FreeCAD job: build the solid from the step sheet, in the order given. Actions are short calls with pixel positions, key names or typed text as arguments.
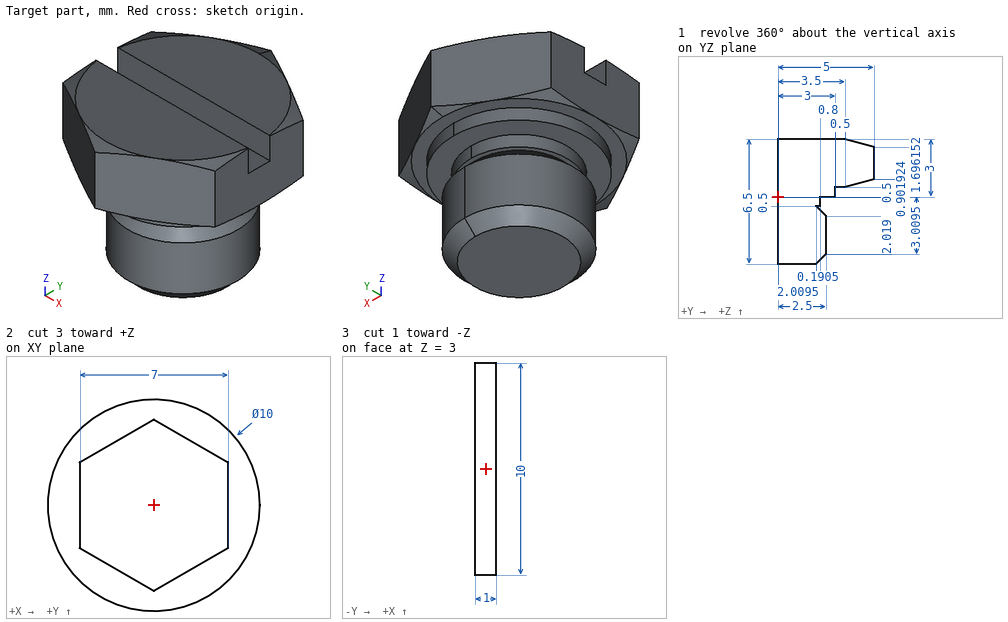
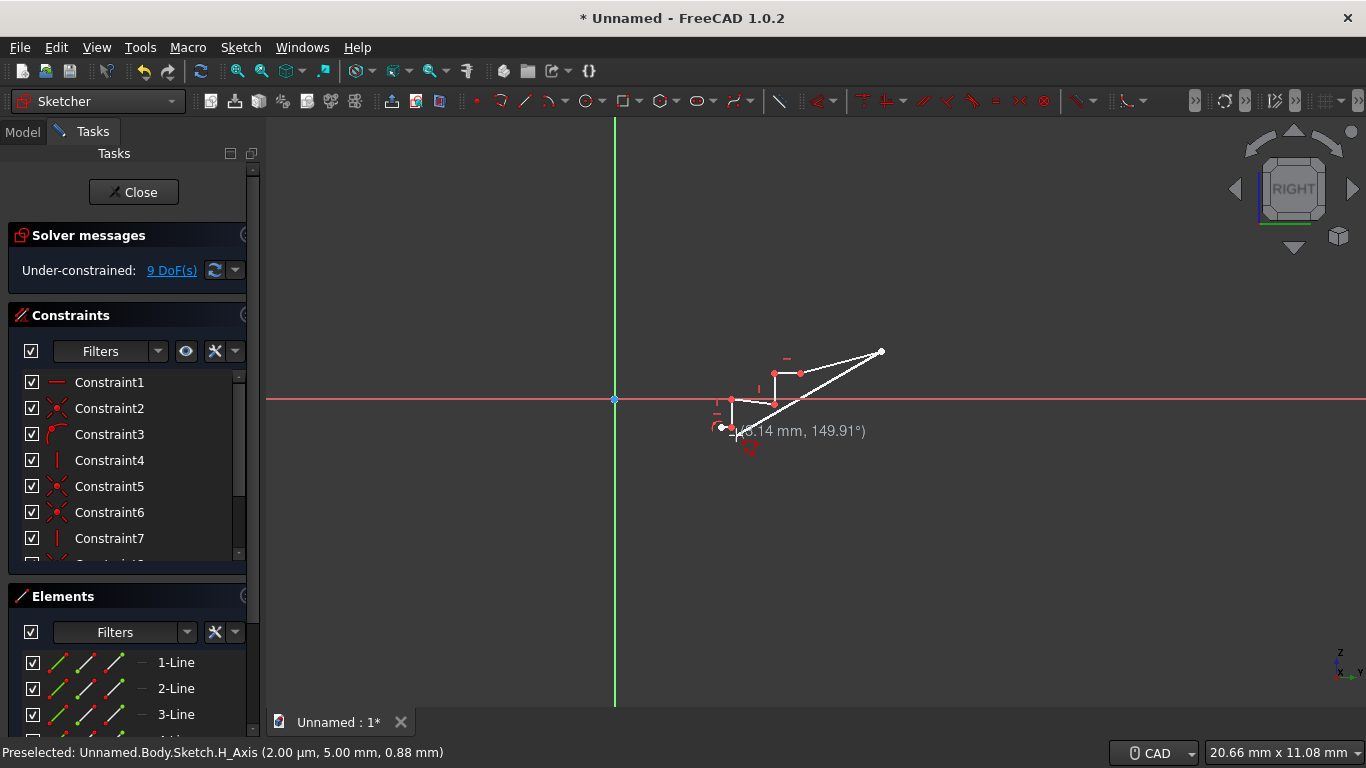
click(881, 261)
click(801, 239)
click(615, 239)
click(624, 586)
click(722, 586)
click(748, 559)
click(748, 452)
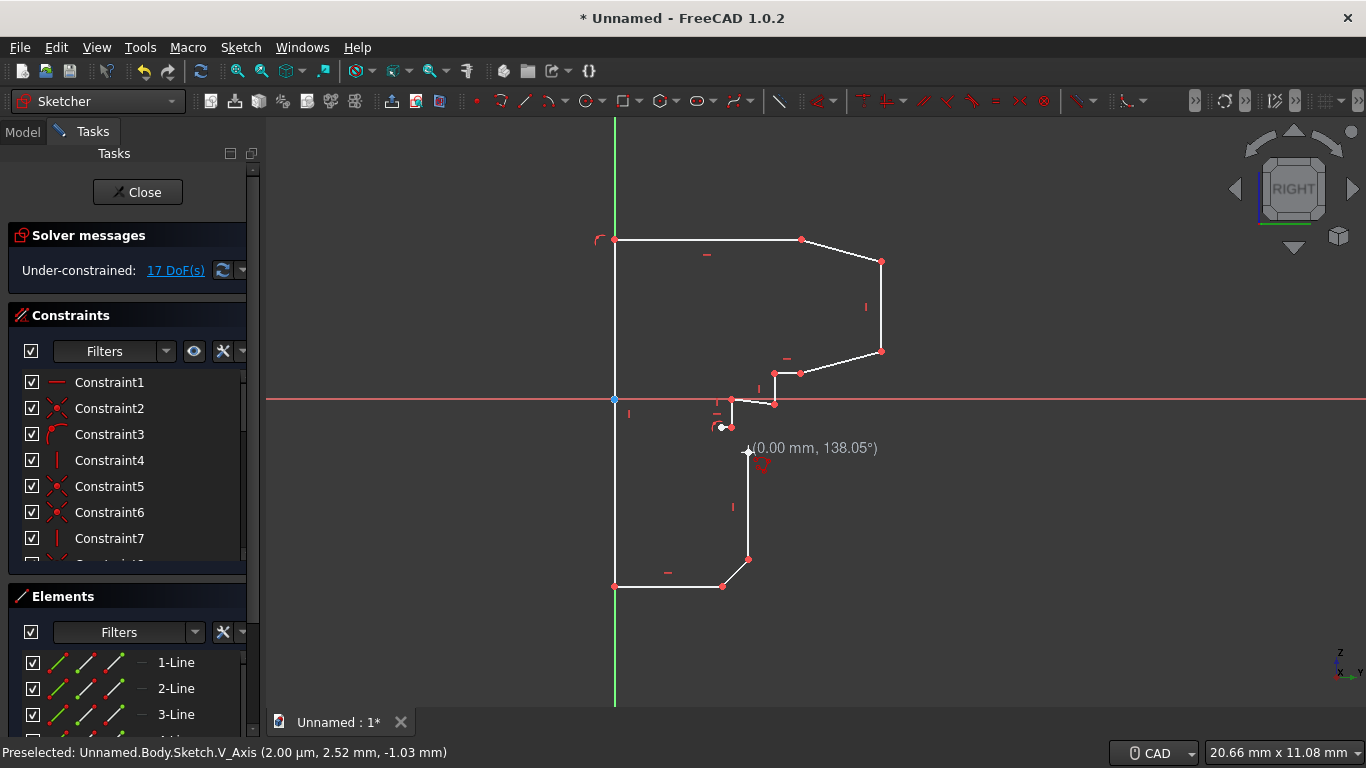
scroll(722, 426, up, 6)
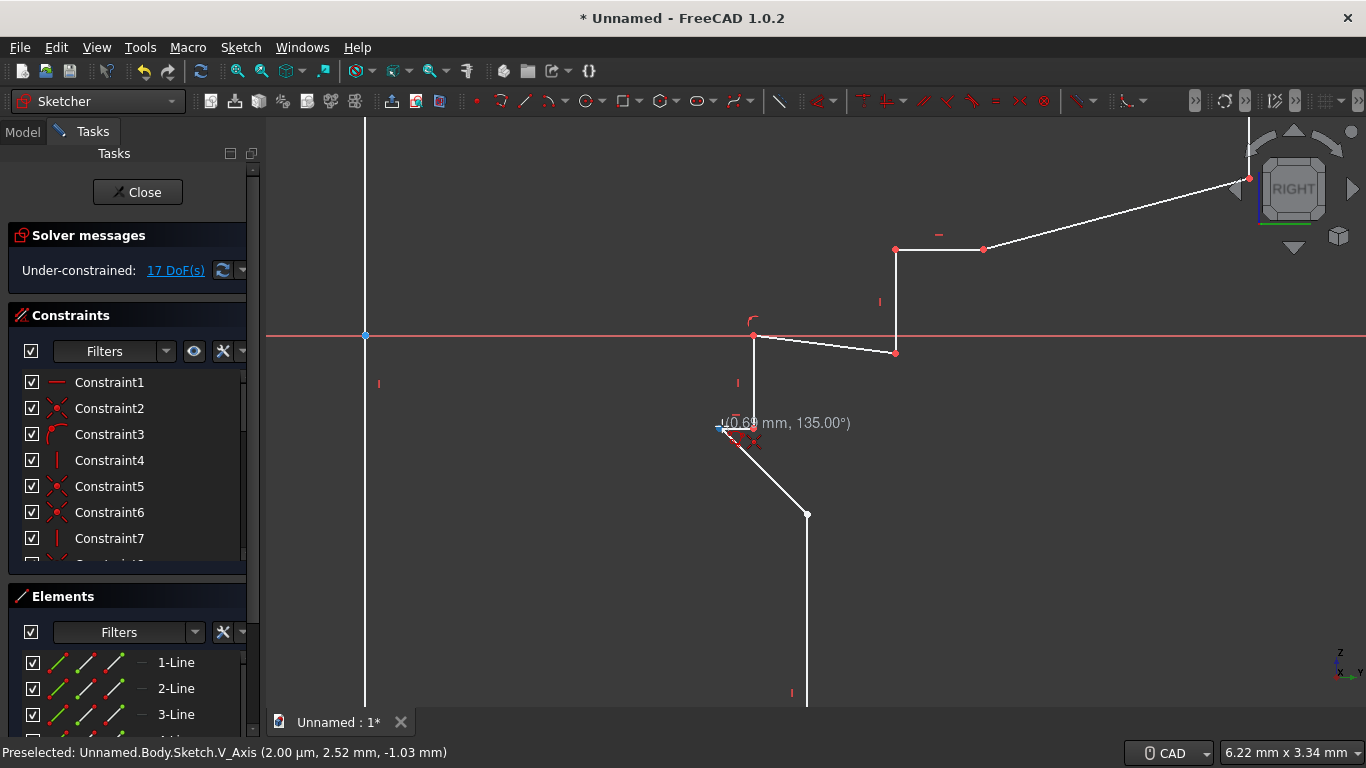
click(720, 429)
key(Escape)
key(Escape)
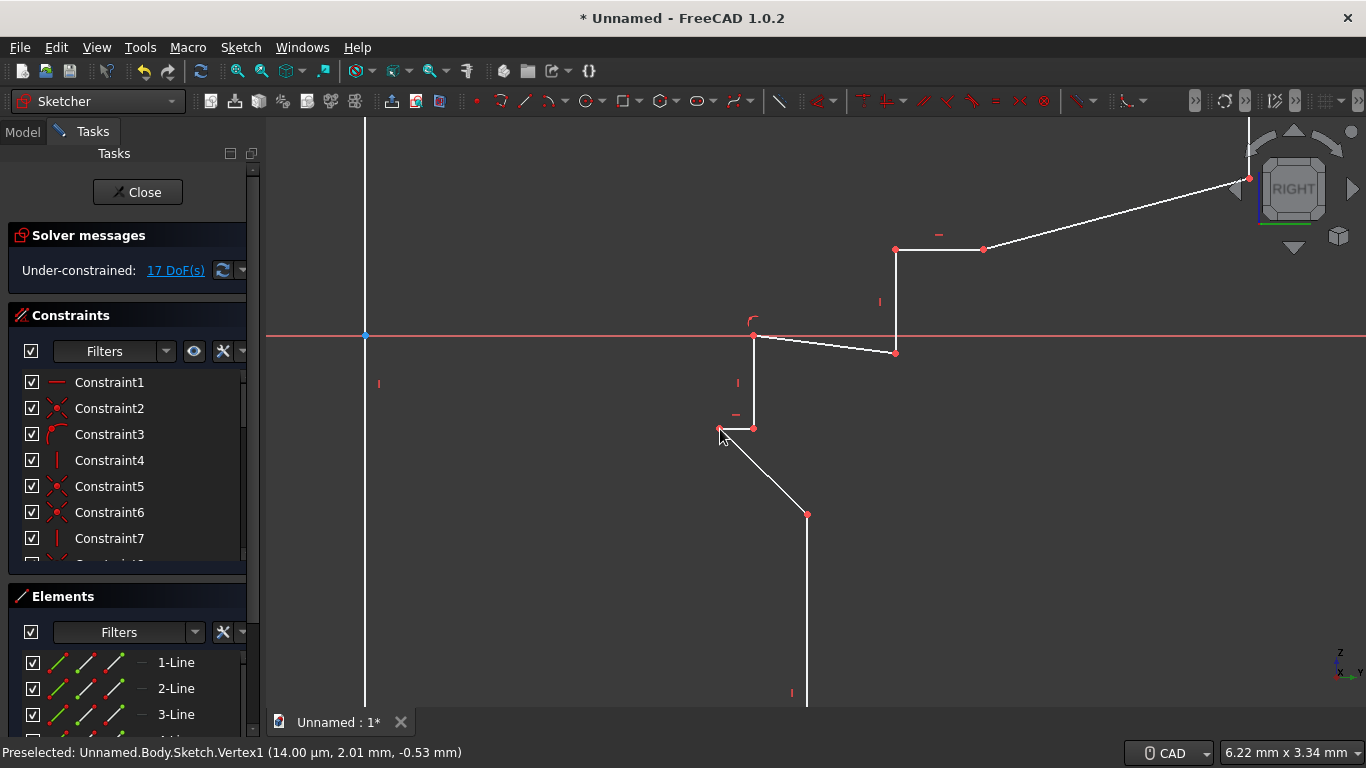
click(853, 348)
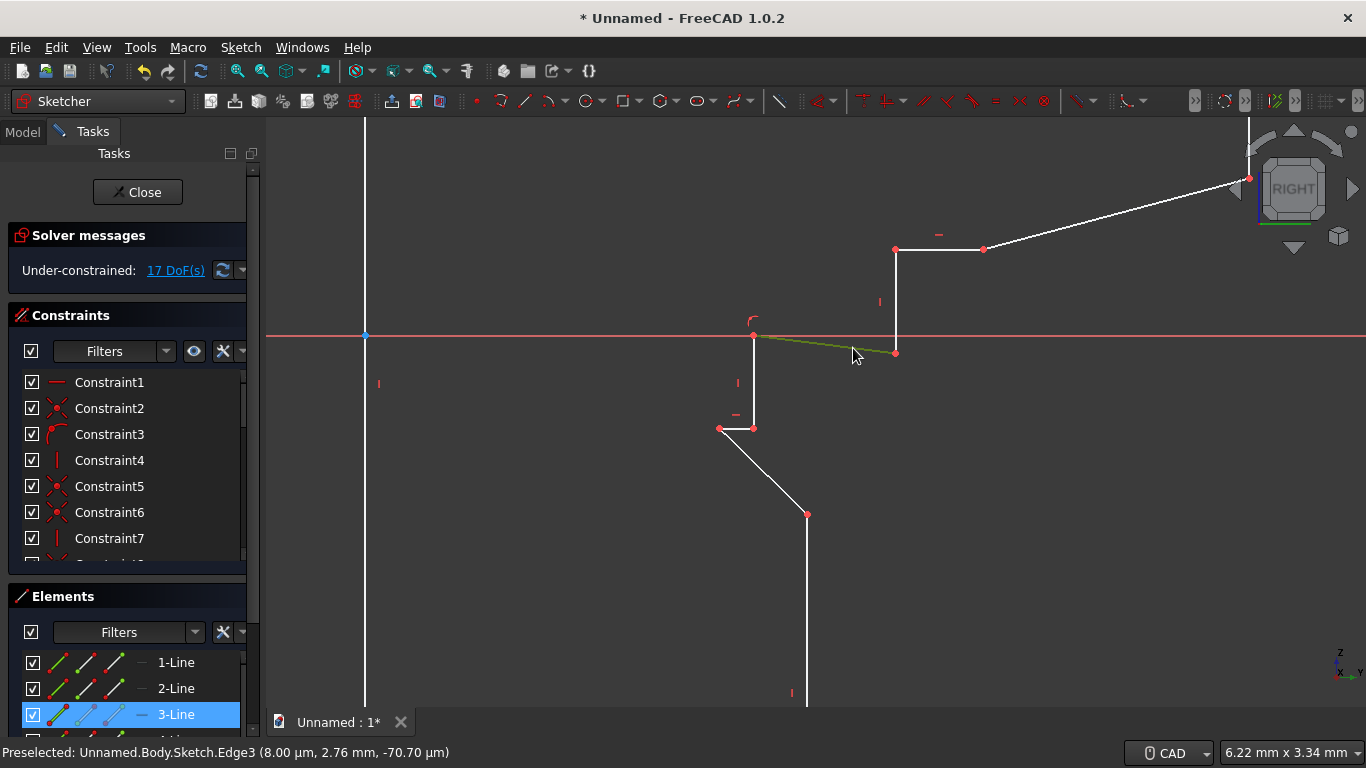
click(906, 102)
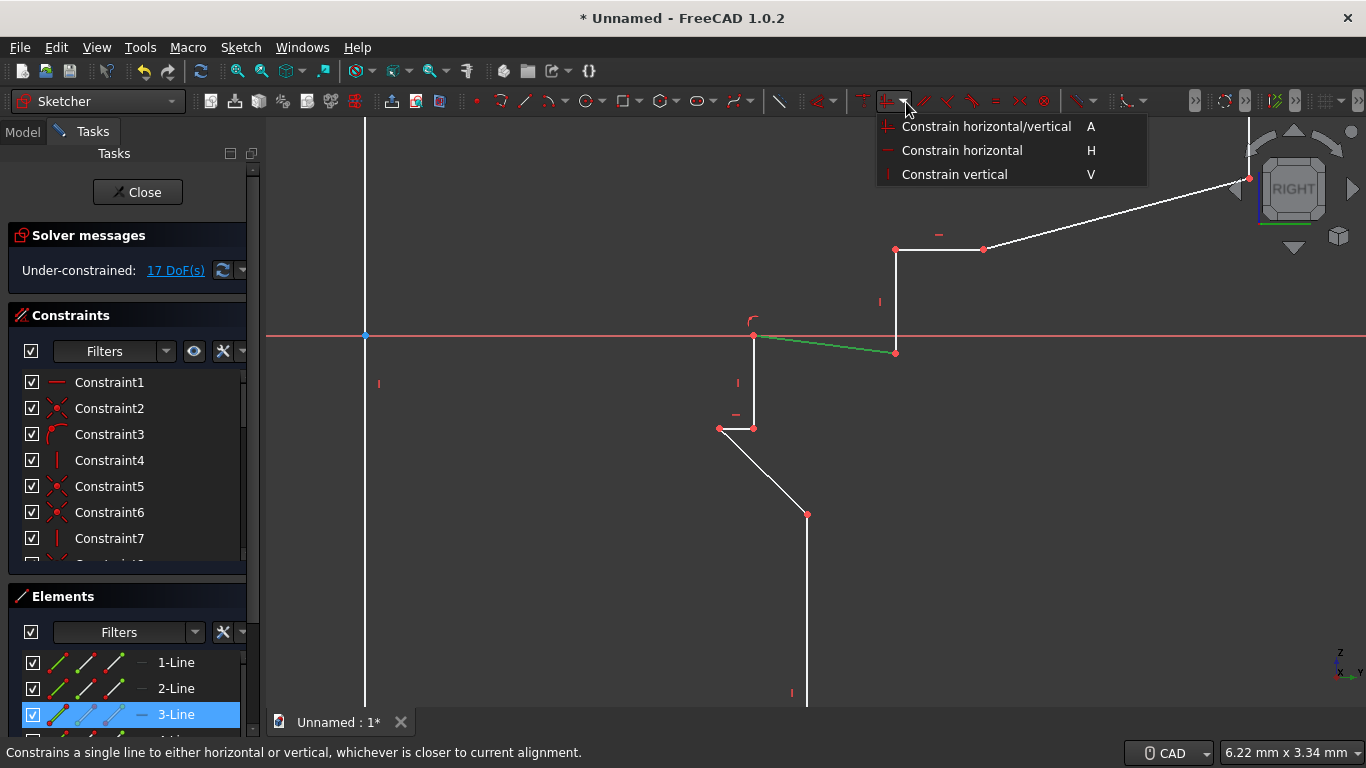
click(1012, 150)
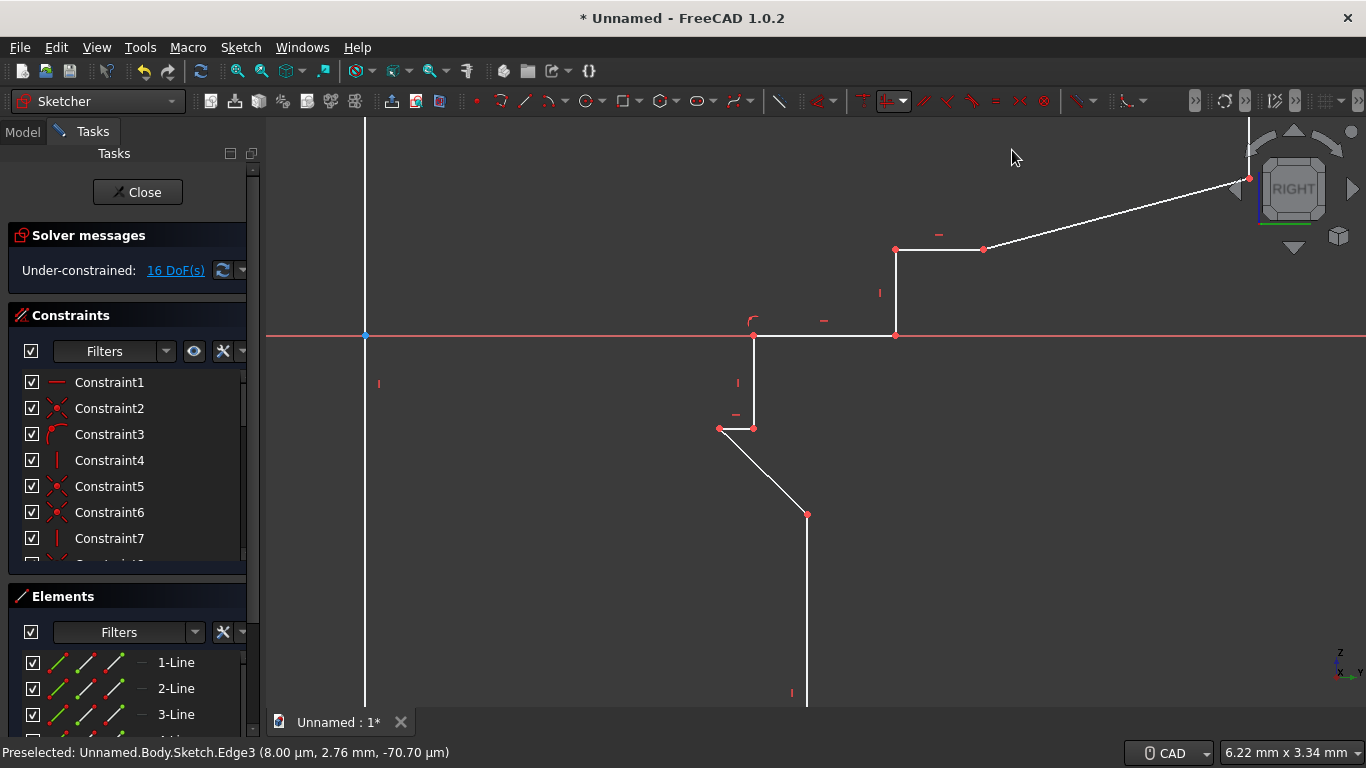
click(818, 102)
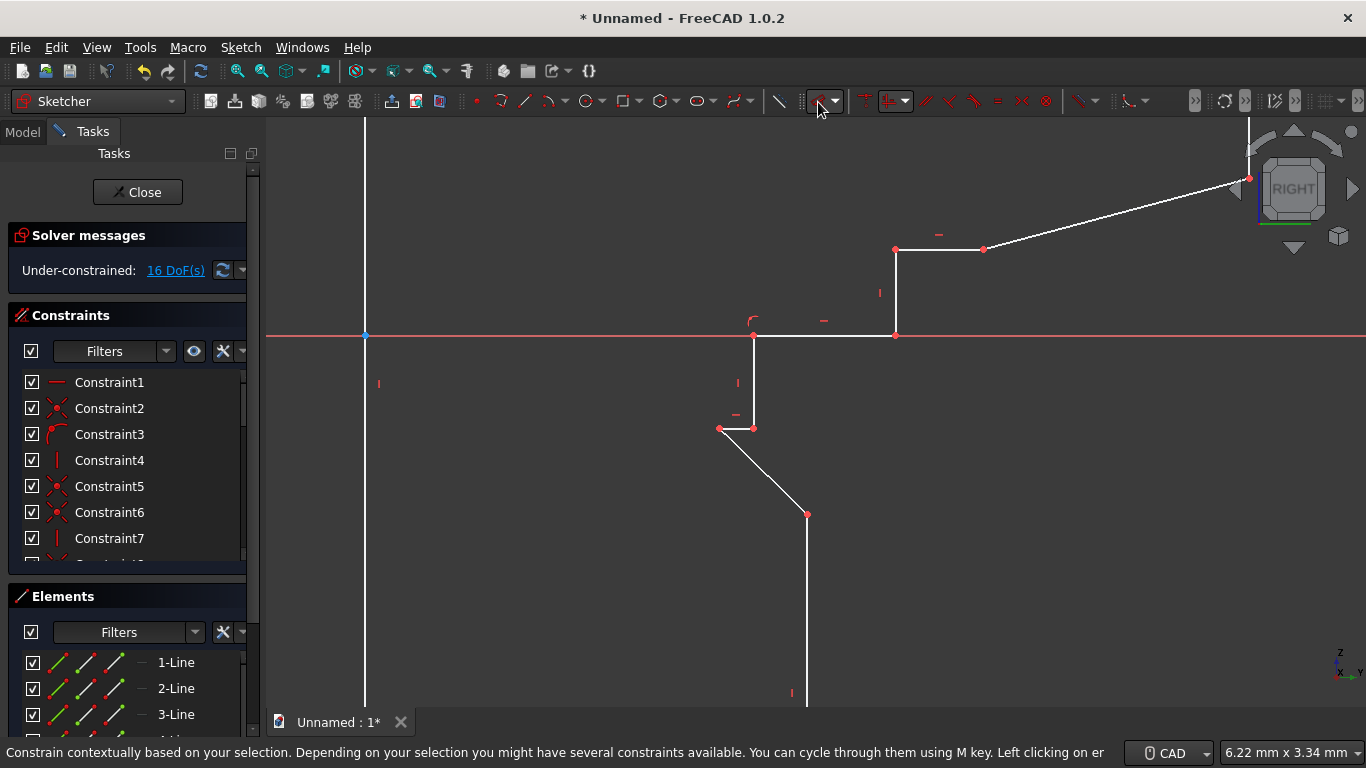
click(896, 336)
click(630, 302)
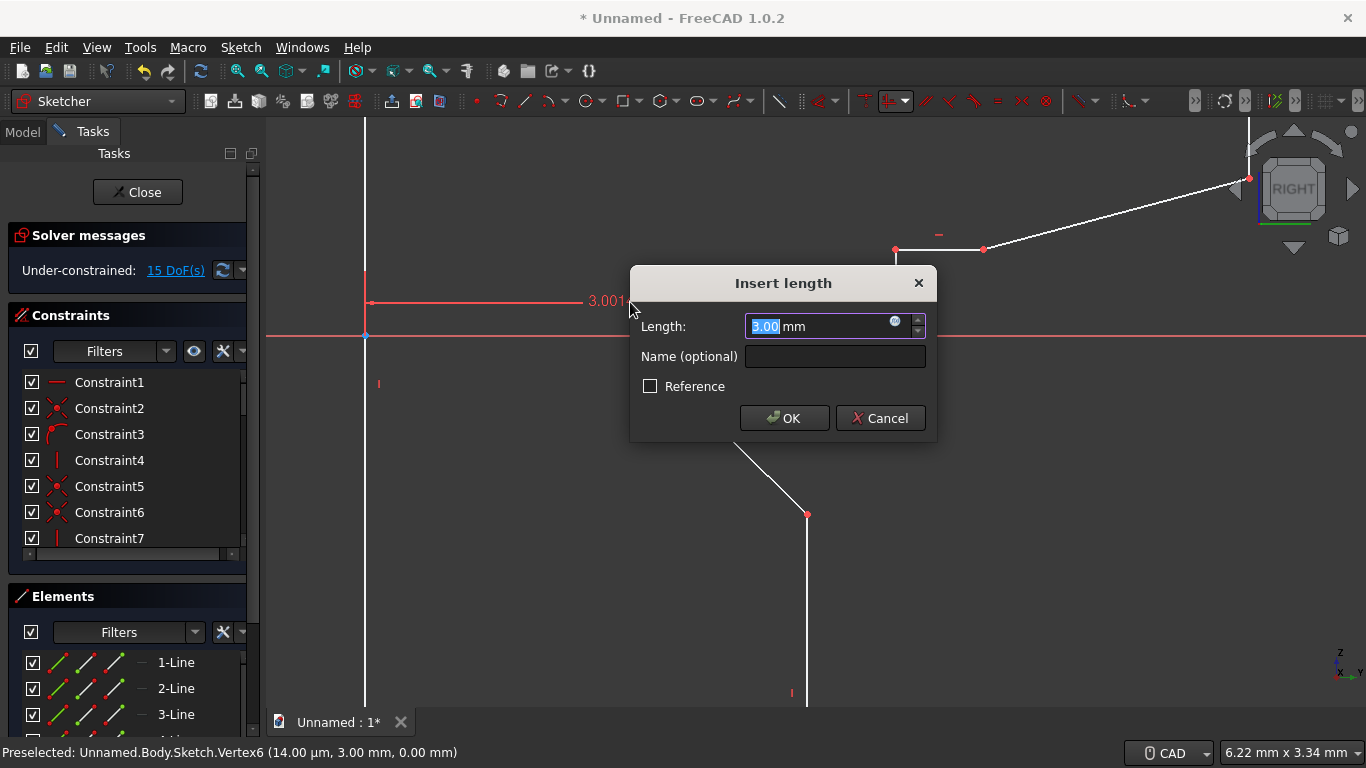
text(3)
key(Return)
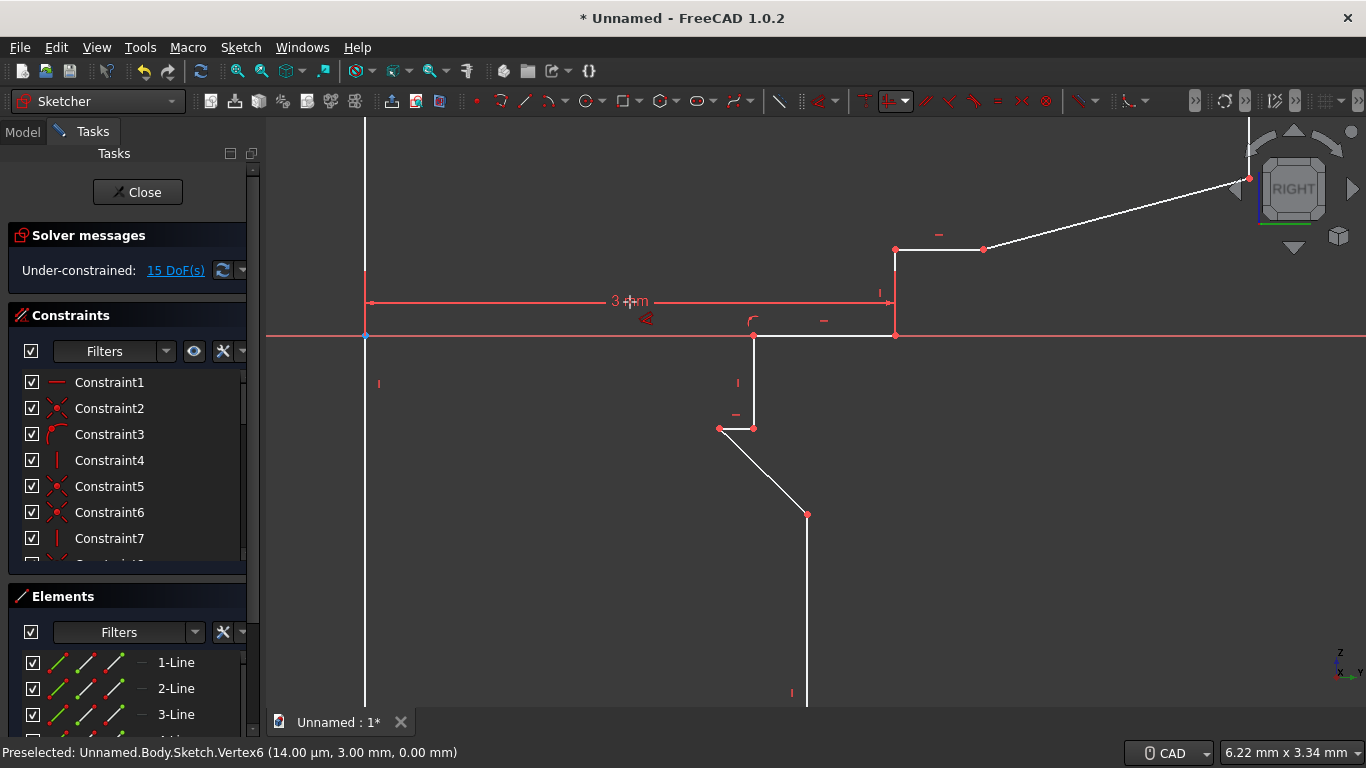
scroll(722, 426, down, 6)